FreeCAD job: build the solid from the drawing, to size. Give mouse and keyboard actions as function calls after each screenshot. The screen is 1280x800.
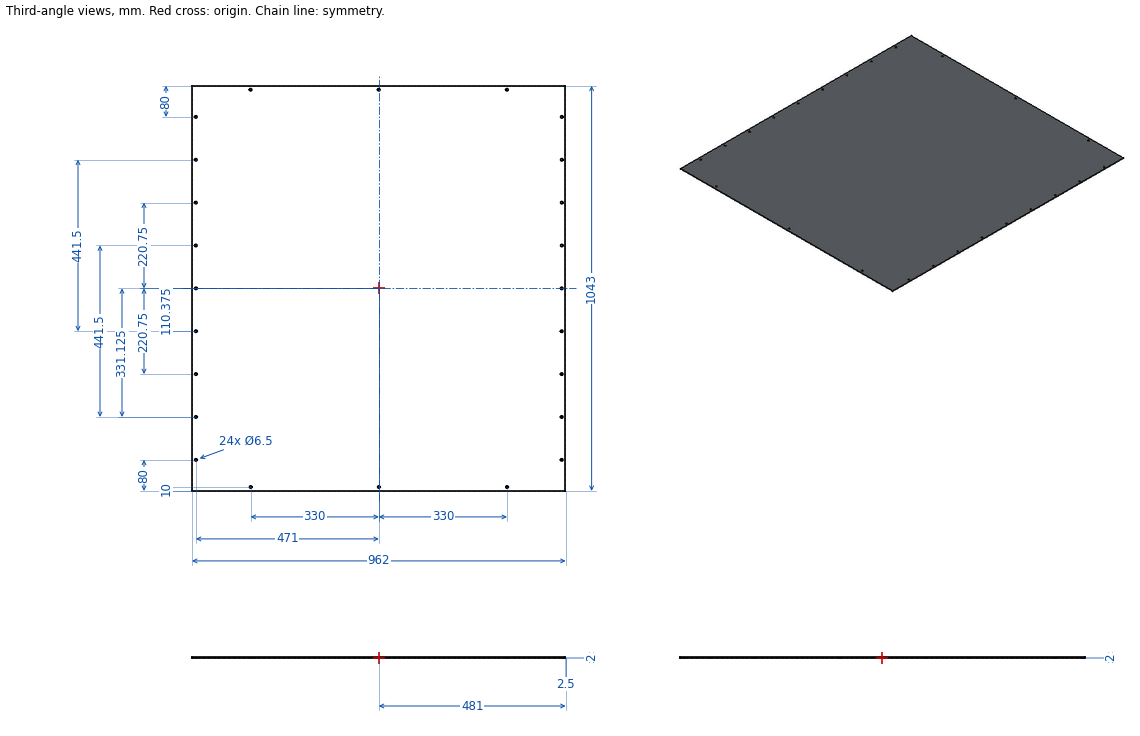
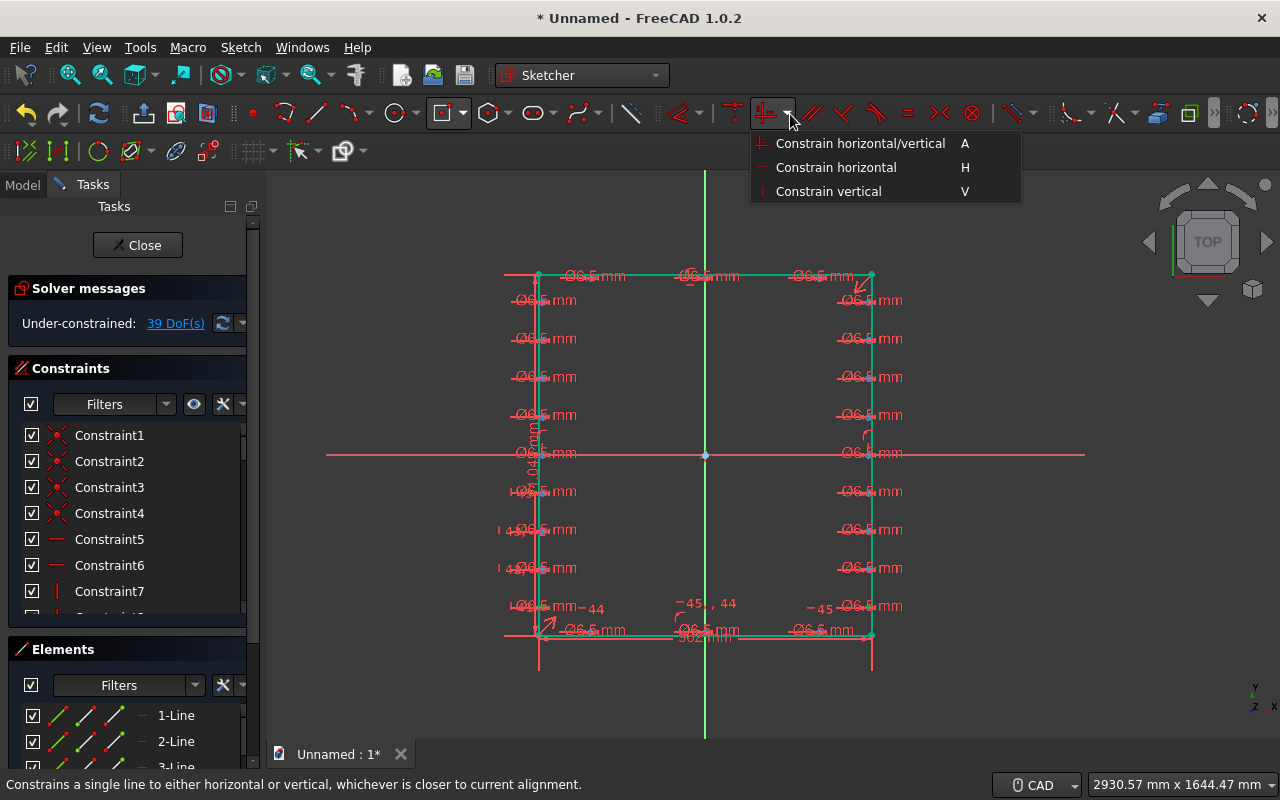
click(886, 167)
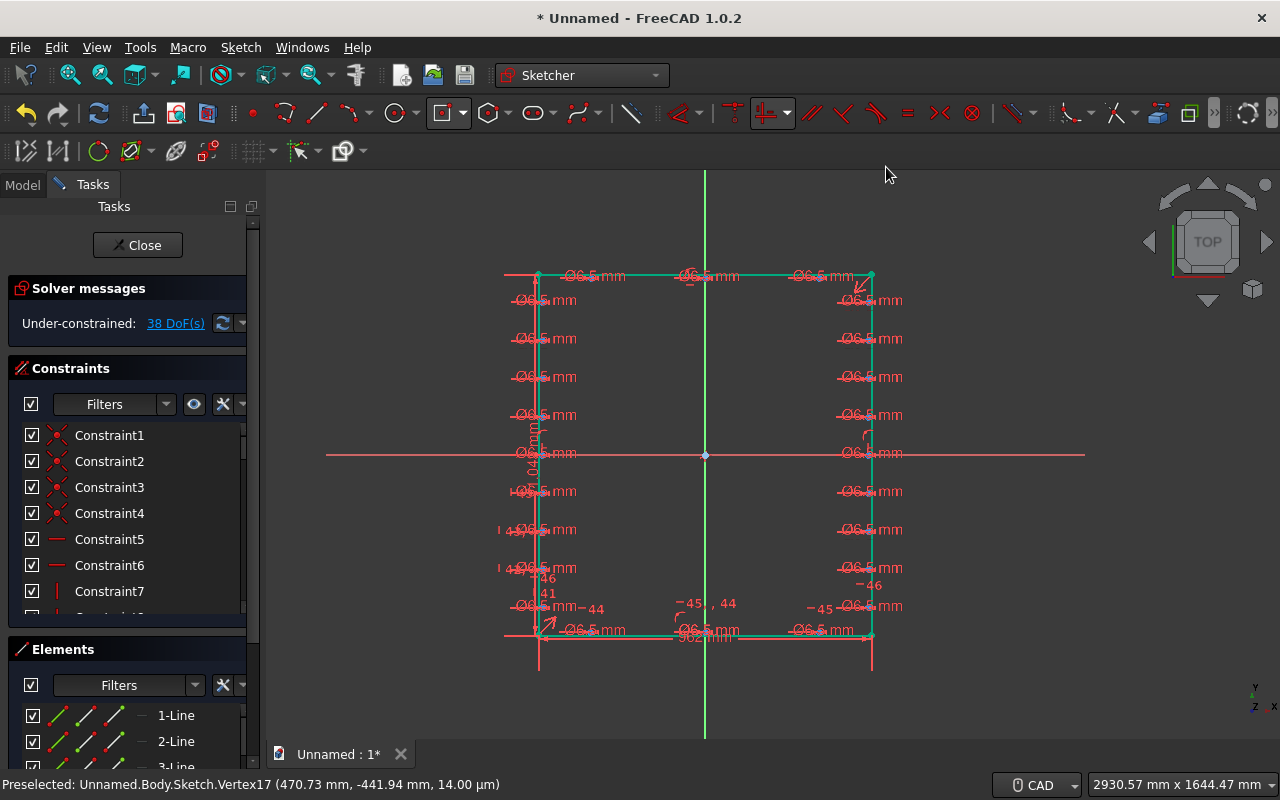
click(868, 608)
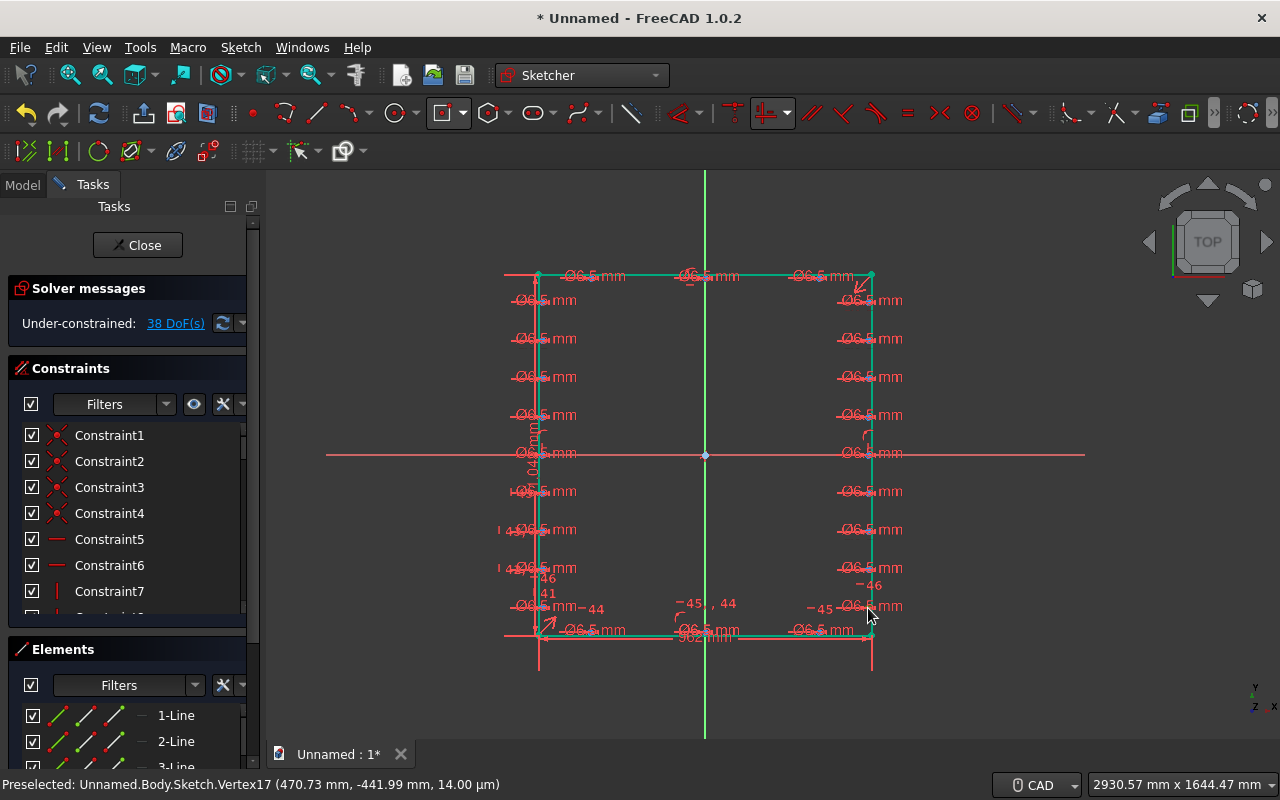
click(868, 570)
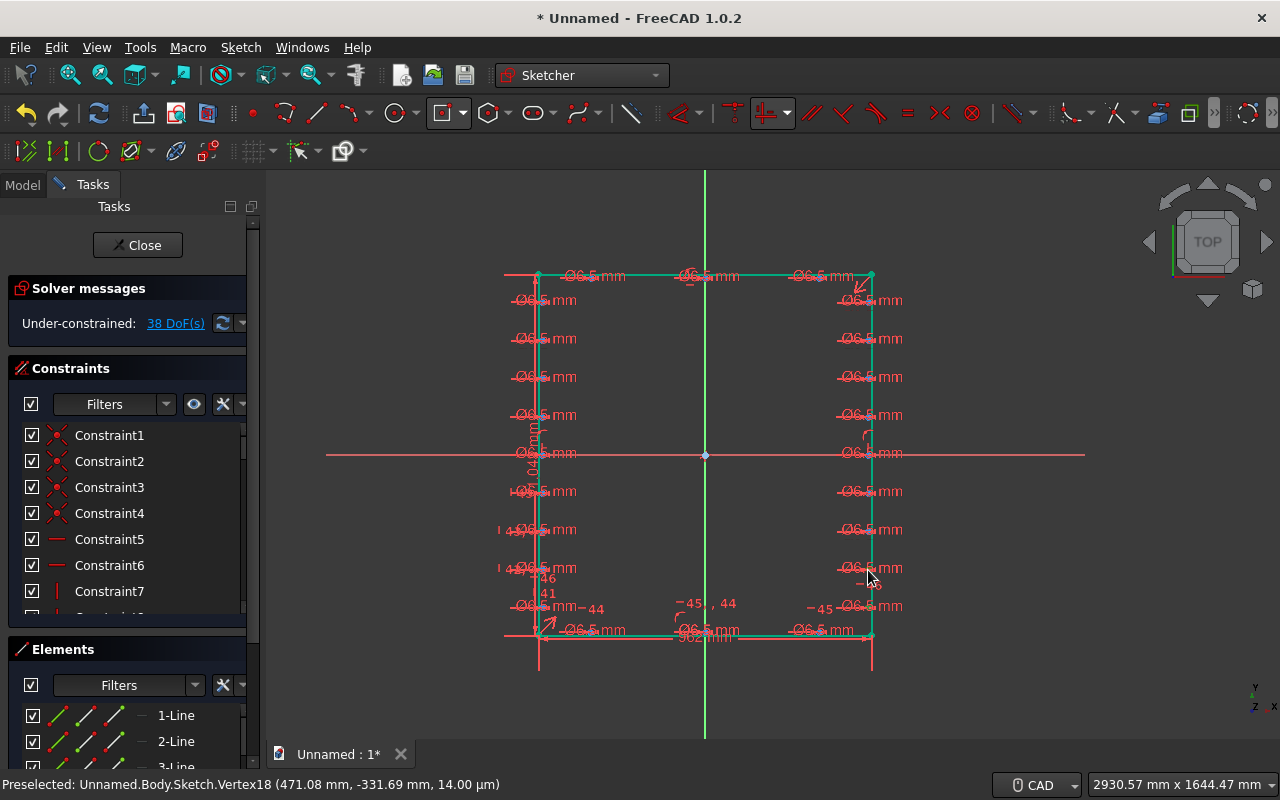
key(v)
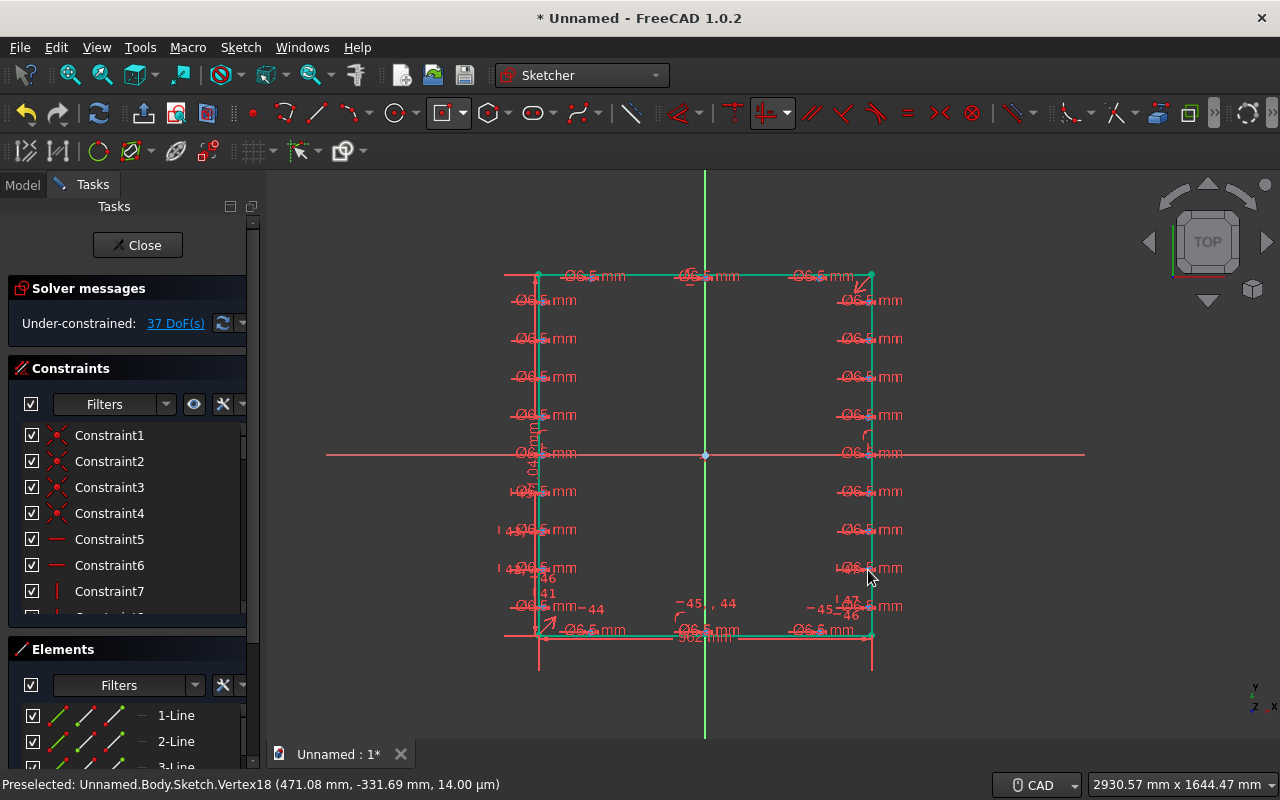
click(868, 570)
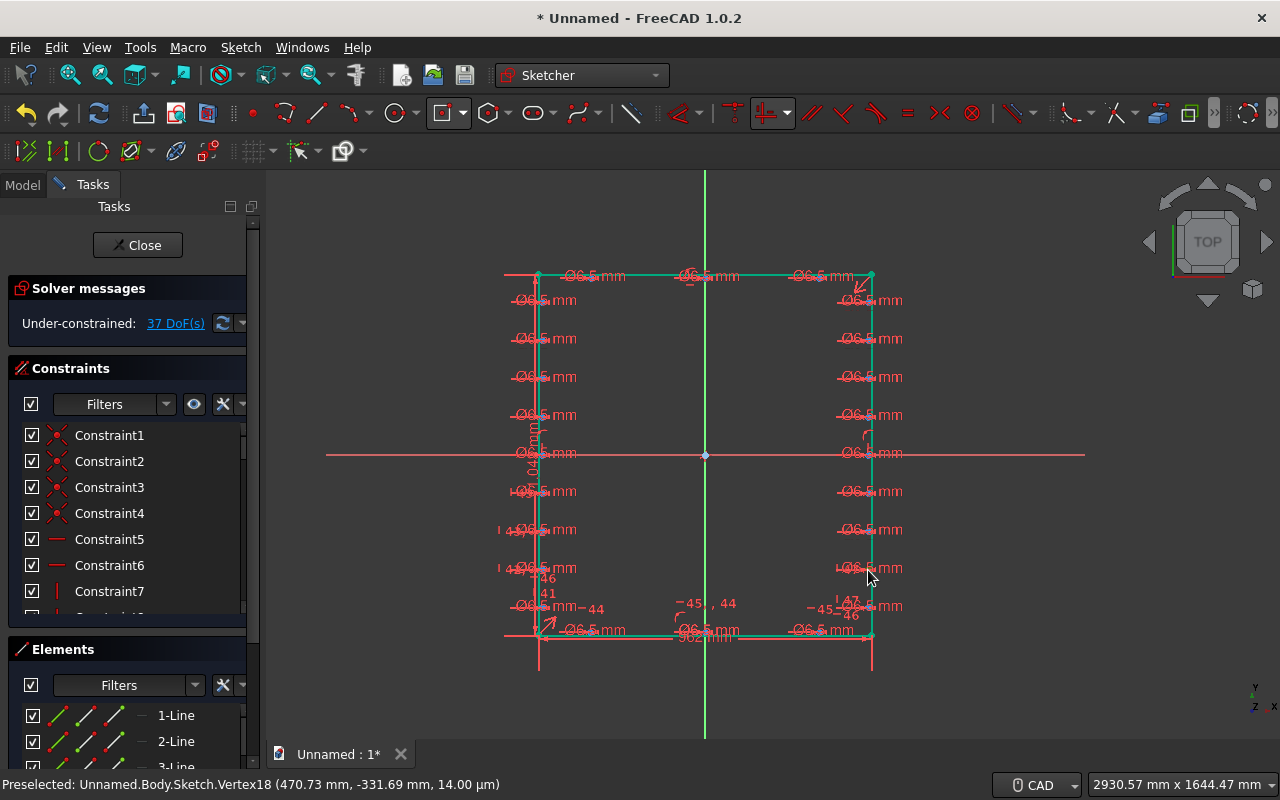
click(868, 532)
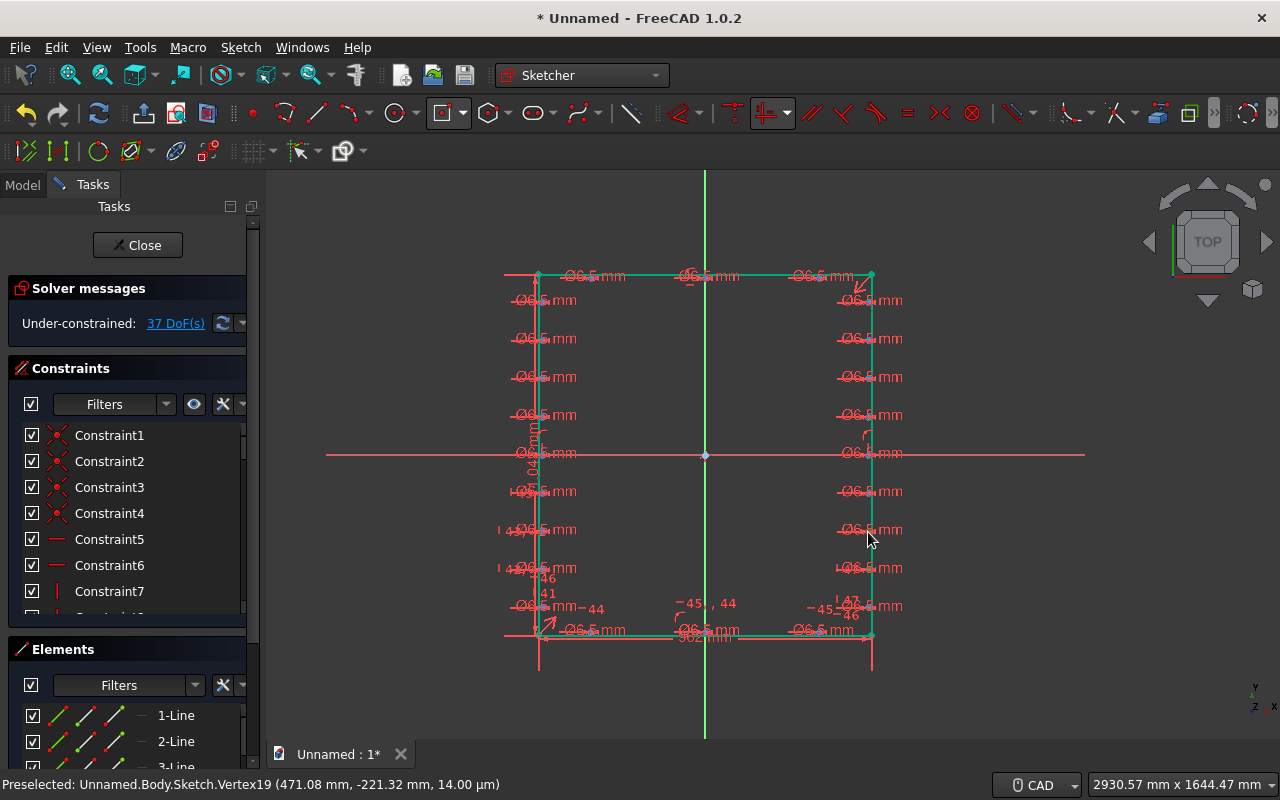
key(v)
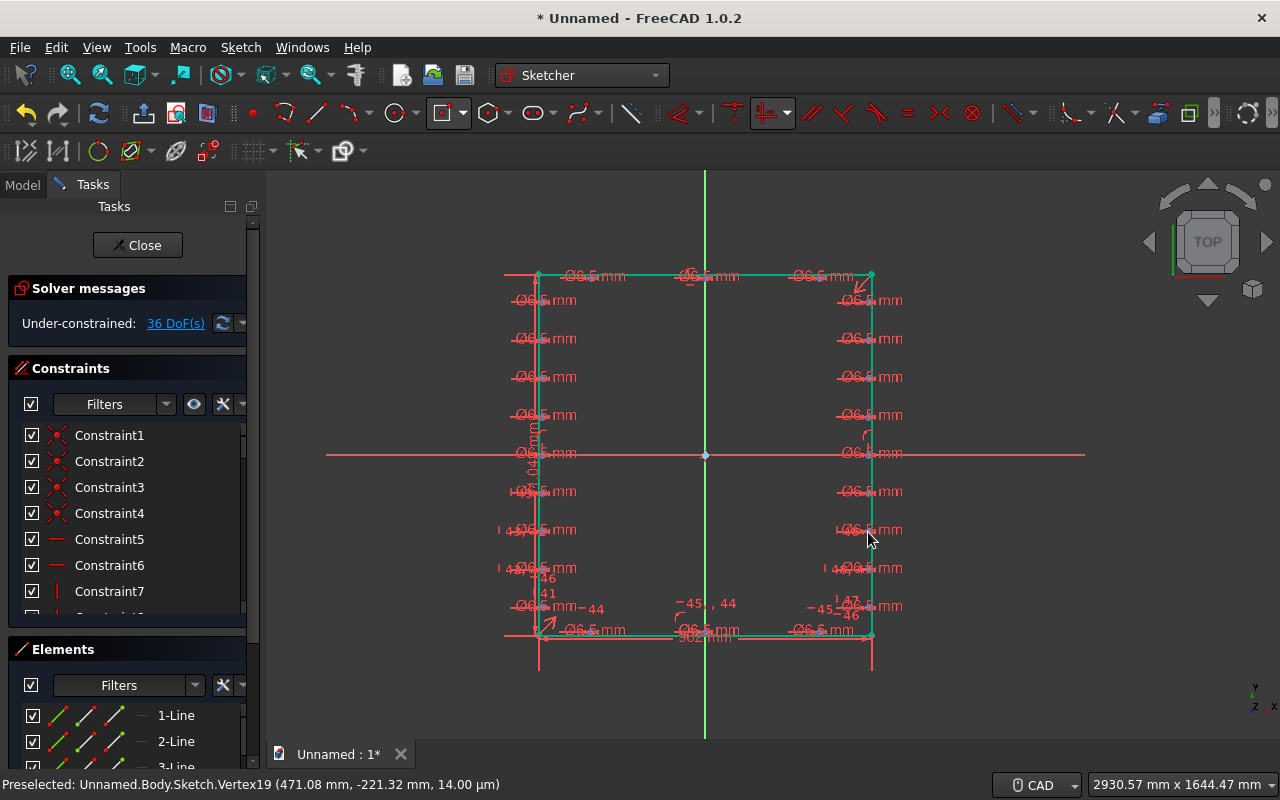
click(868, 532)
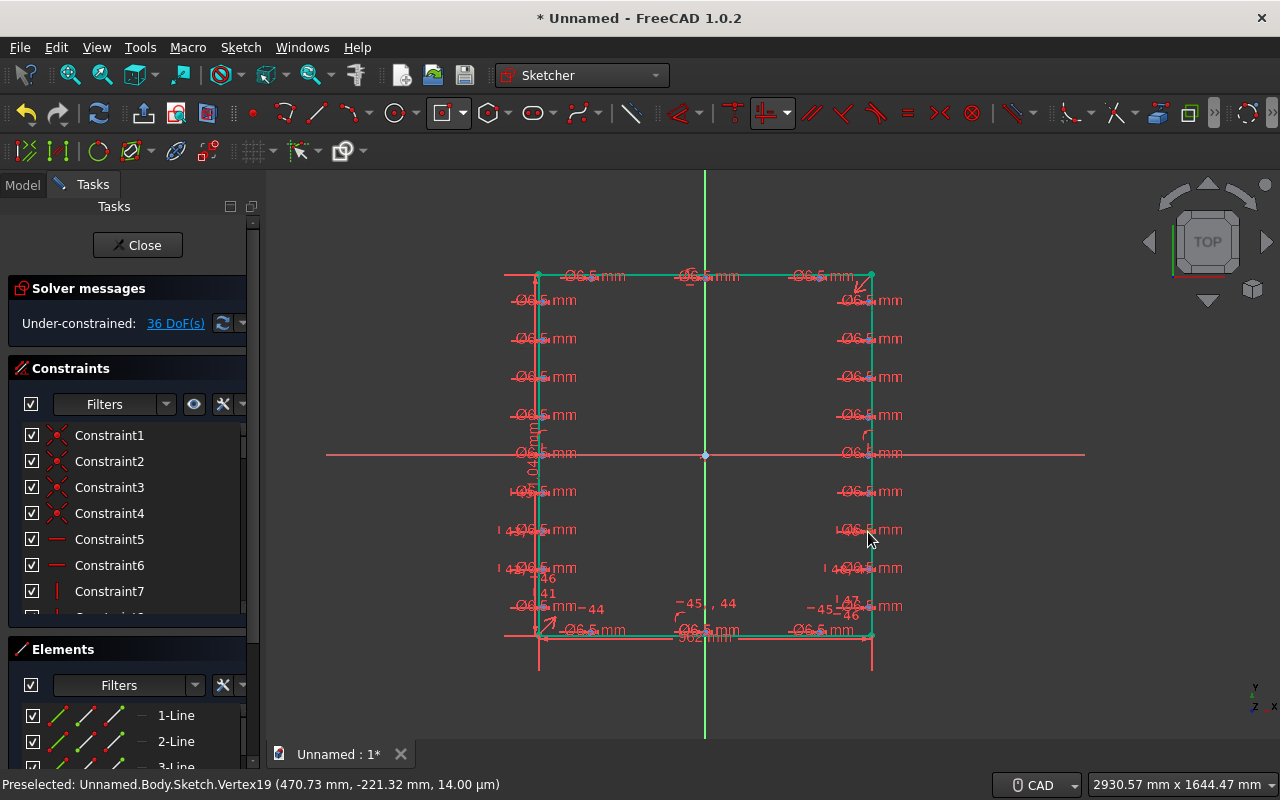
click(868, 493)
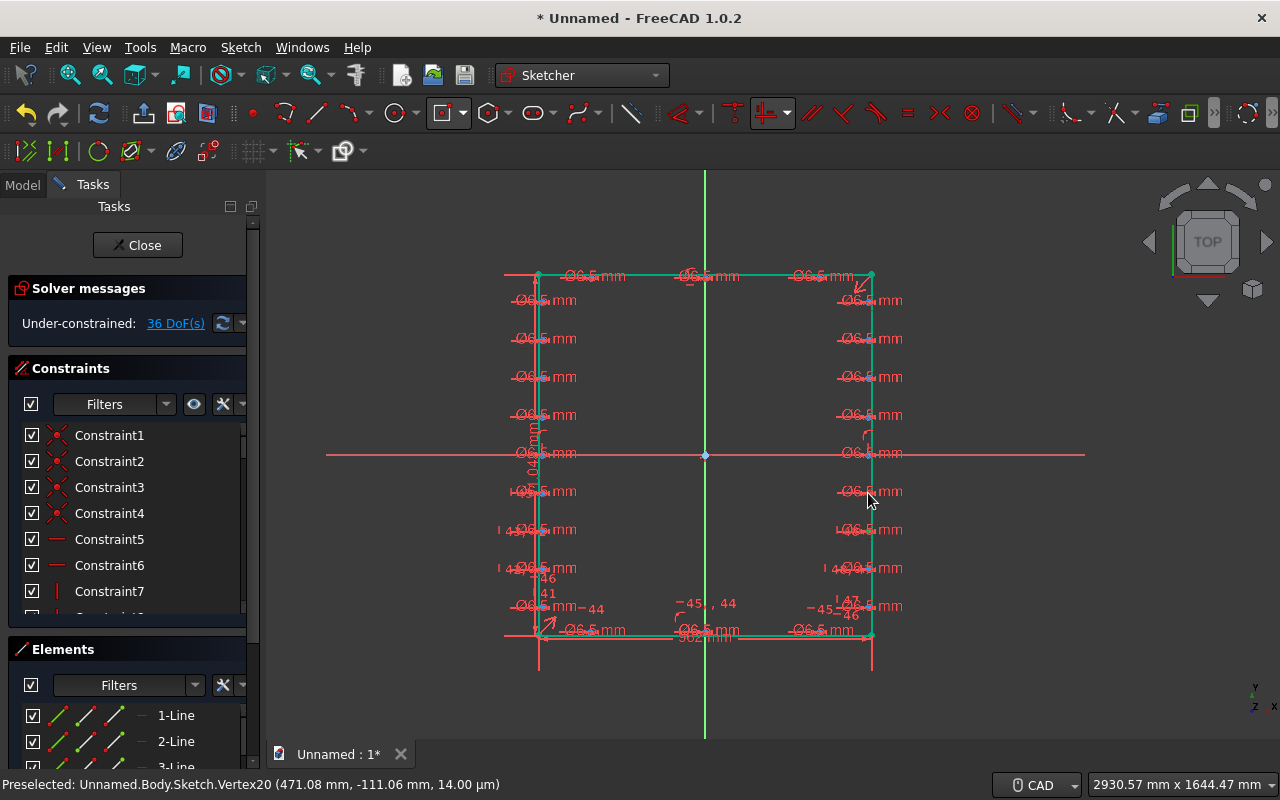
key(v)